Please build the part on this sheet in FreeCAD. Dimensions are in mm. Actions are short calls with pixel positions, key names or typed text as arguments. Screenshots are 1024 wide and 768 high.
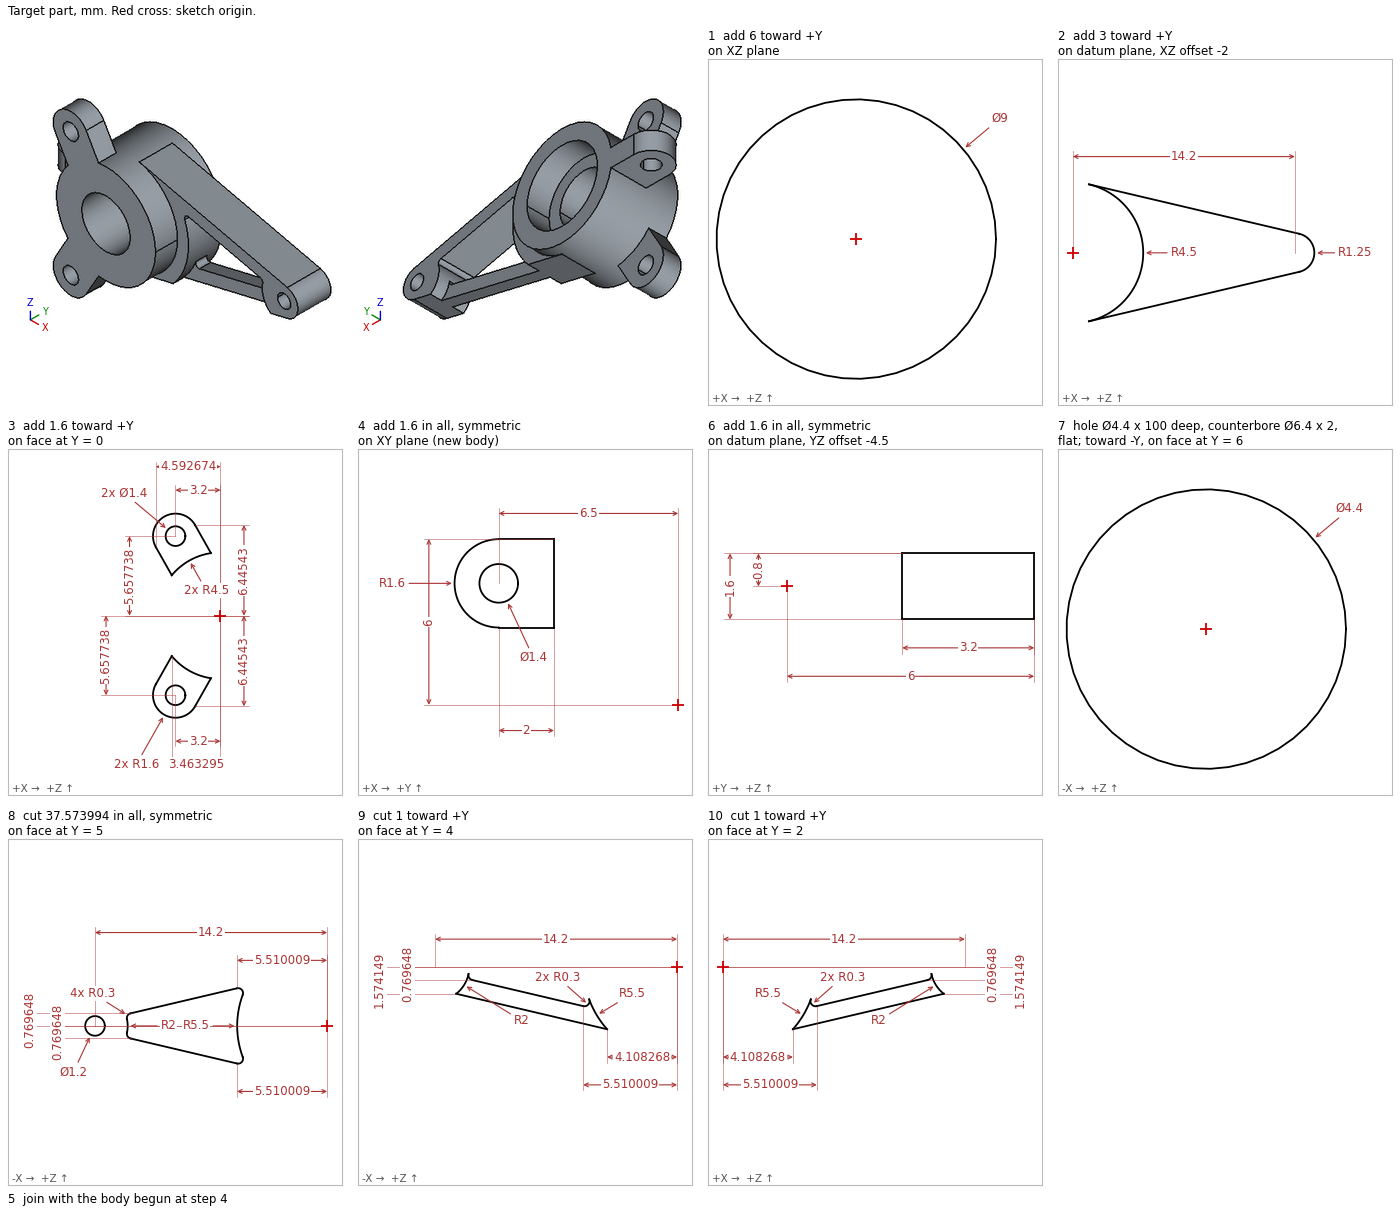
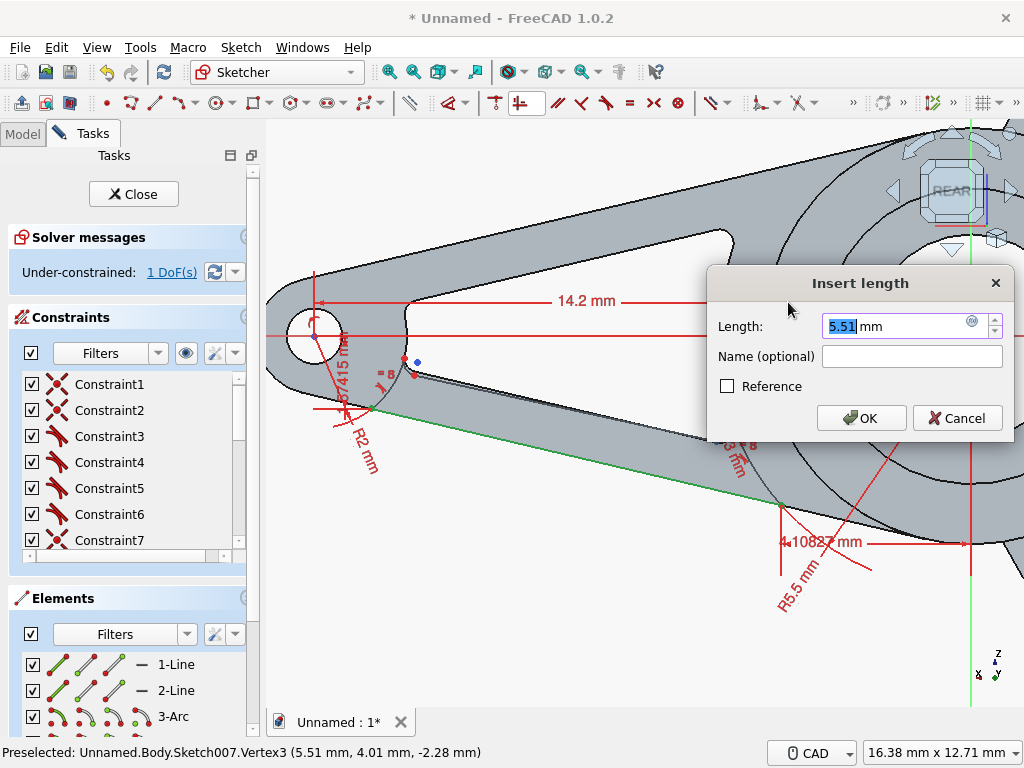
text(5.510009)
key(Return)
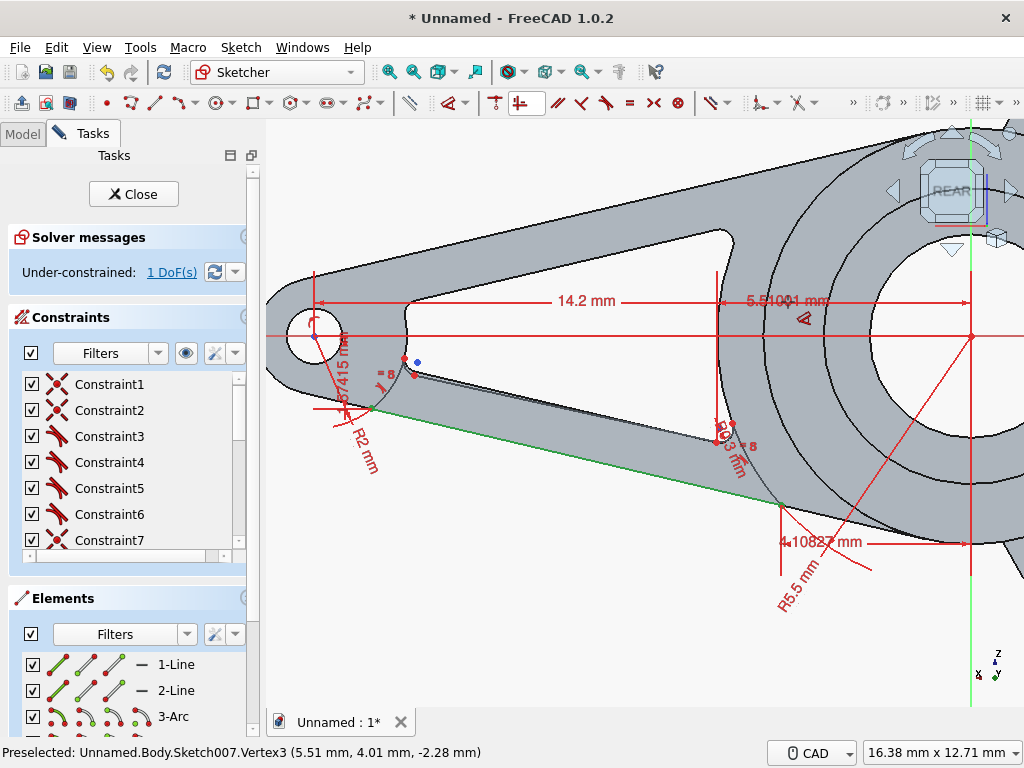
click(415, 376)
click(381, 356)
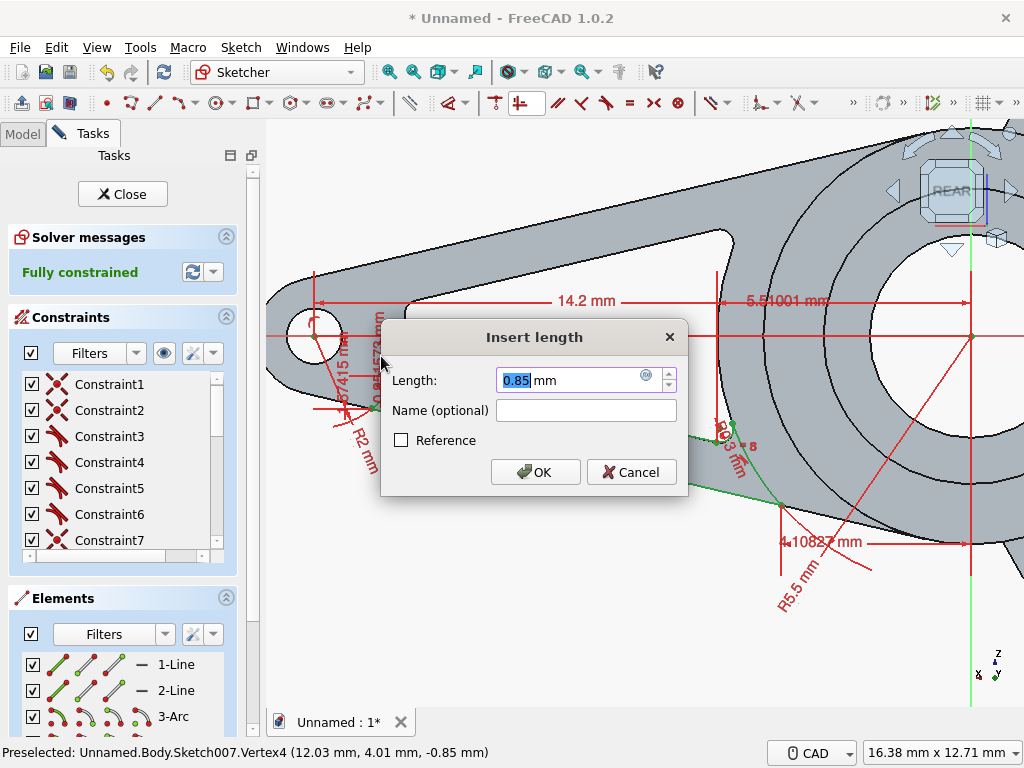
text(0.769648)
key(Return)
key(Escape)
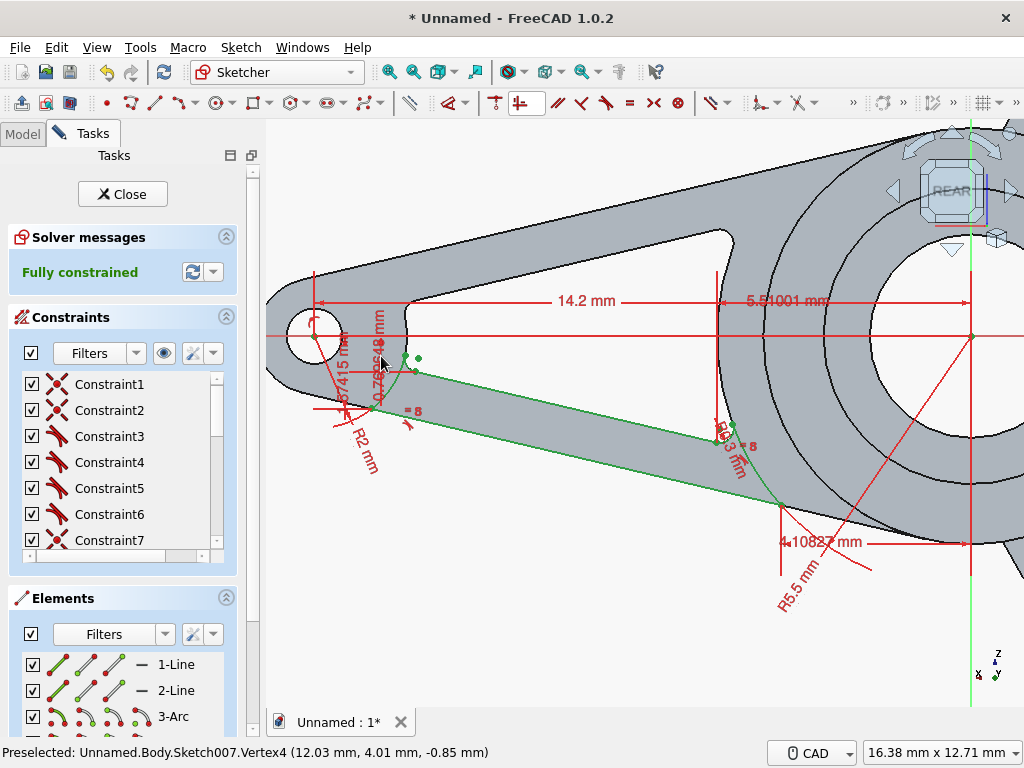
click(123, 194)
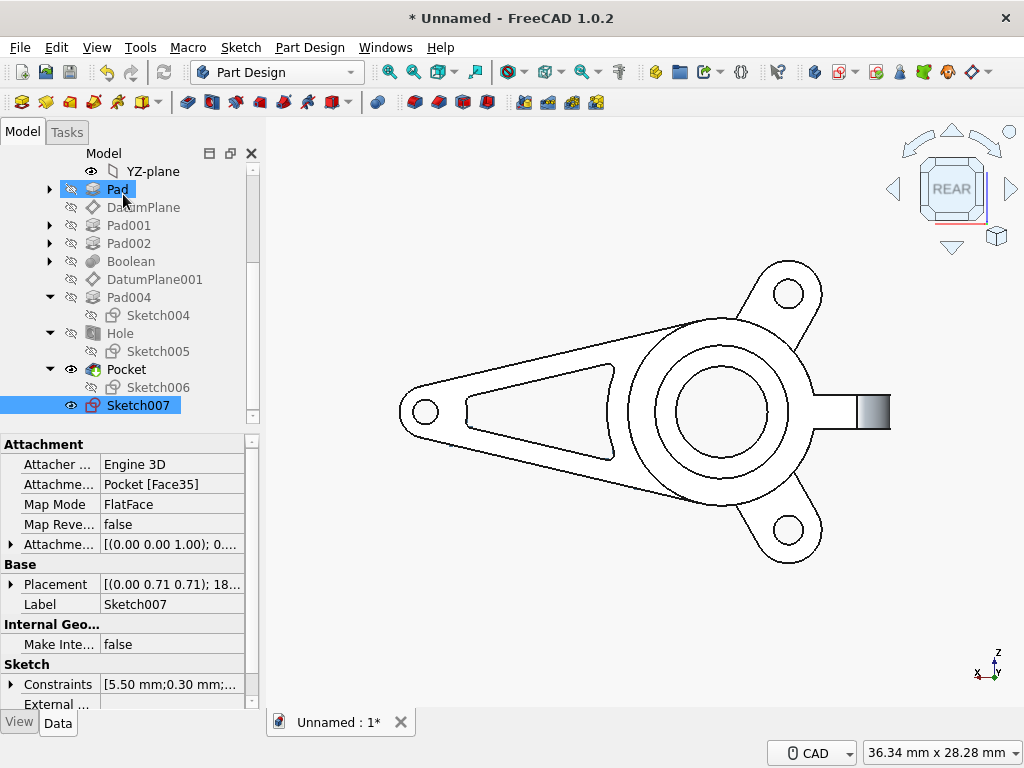
click(188, 102)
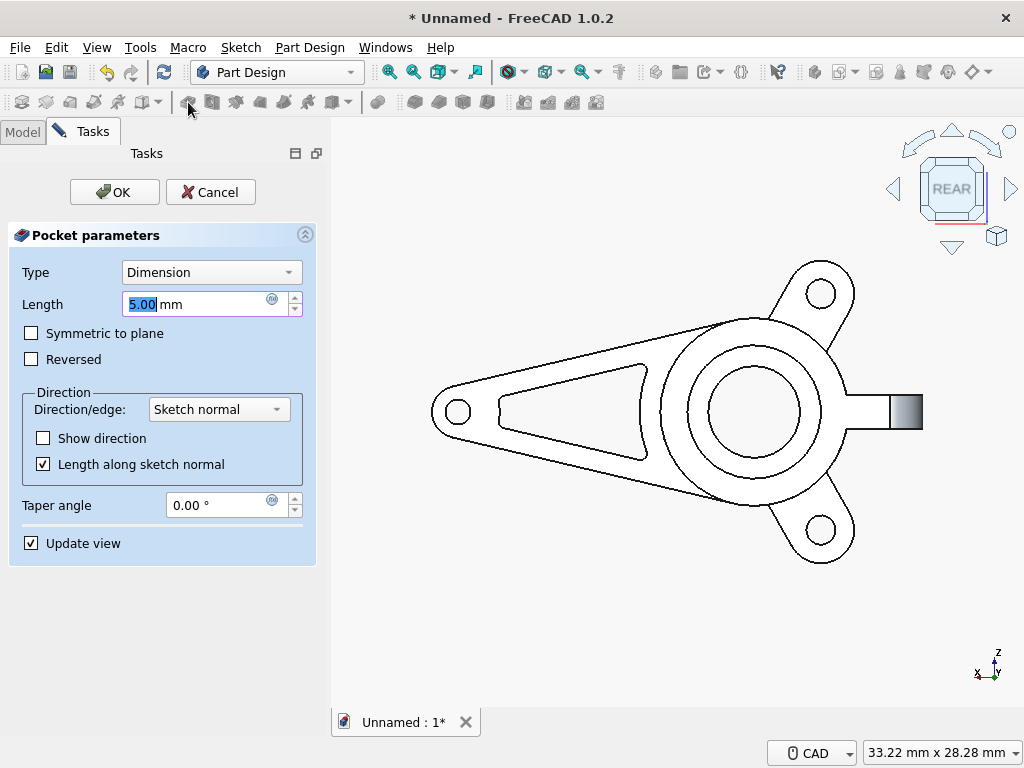
text(1)
key(Tab)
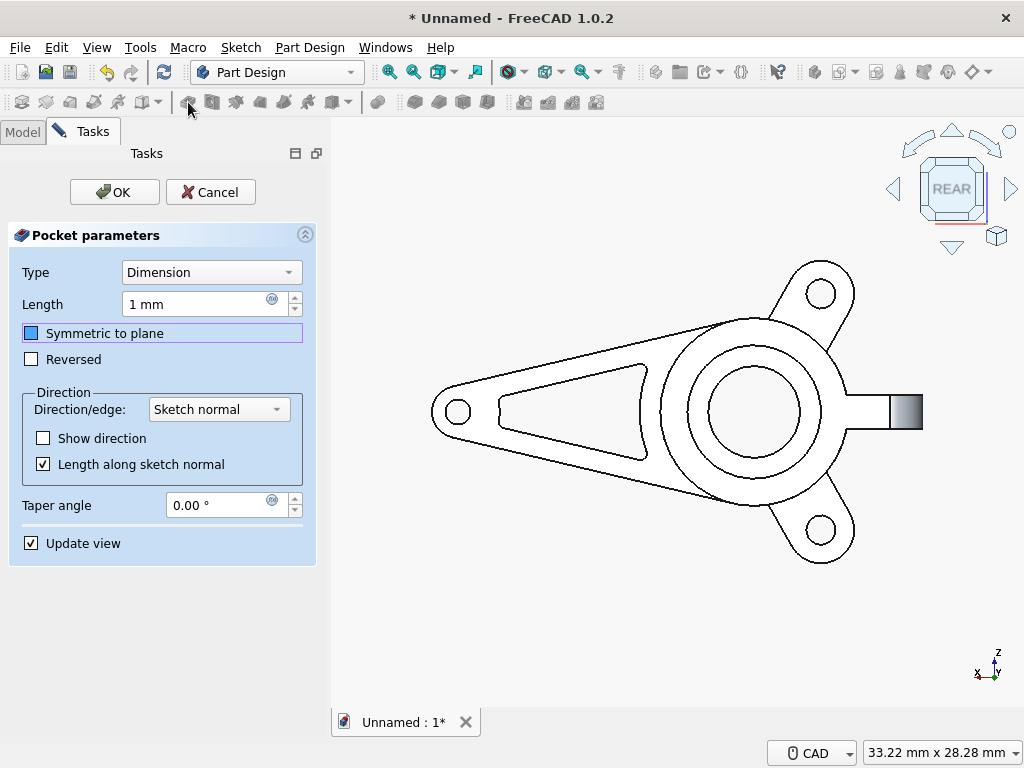
click(30, 359)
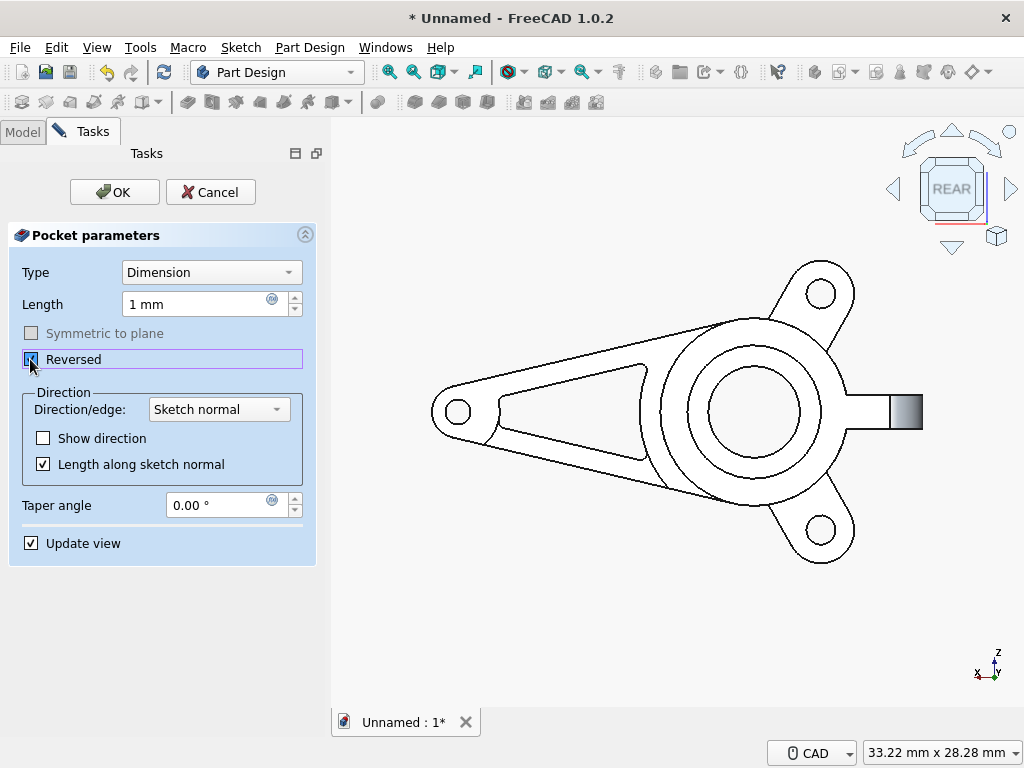
click(115, 192)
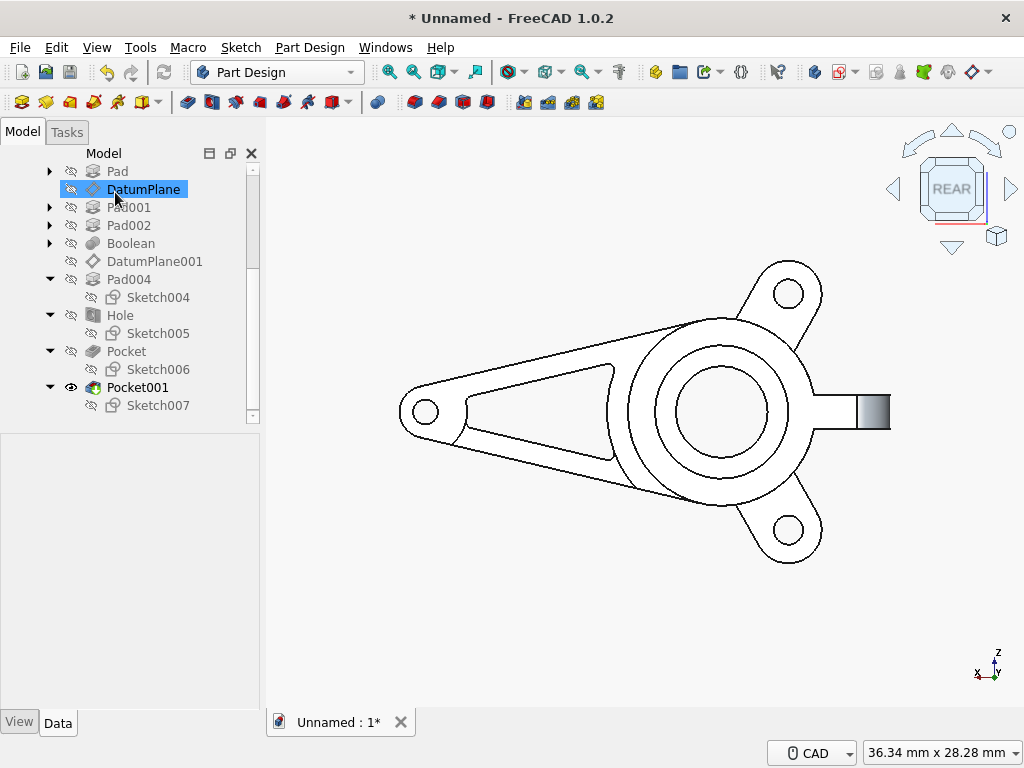
key(0)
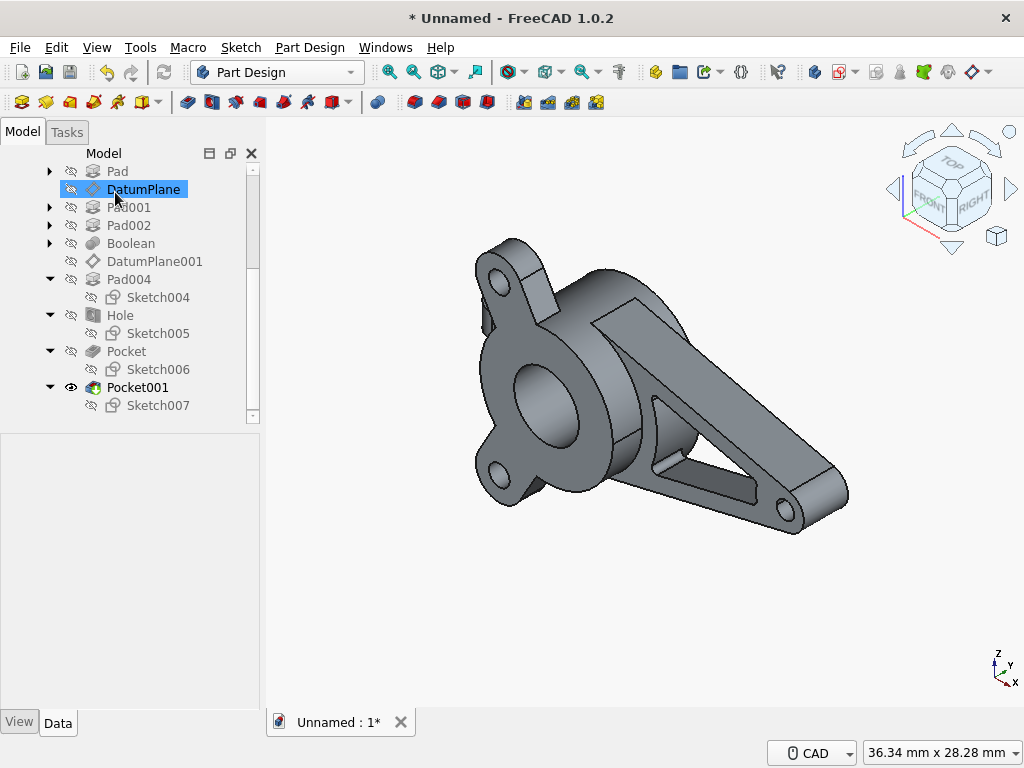
click(758, 515)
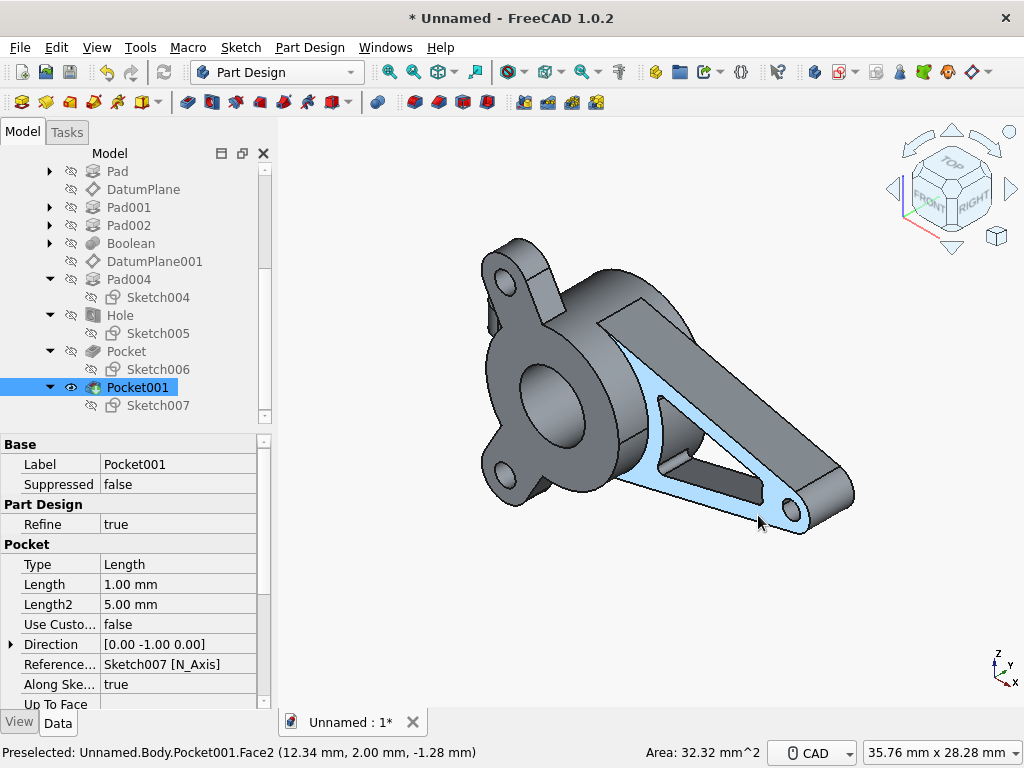
click(840, 72)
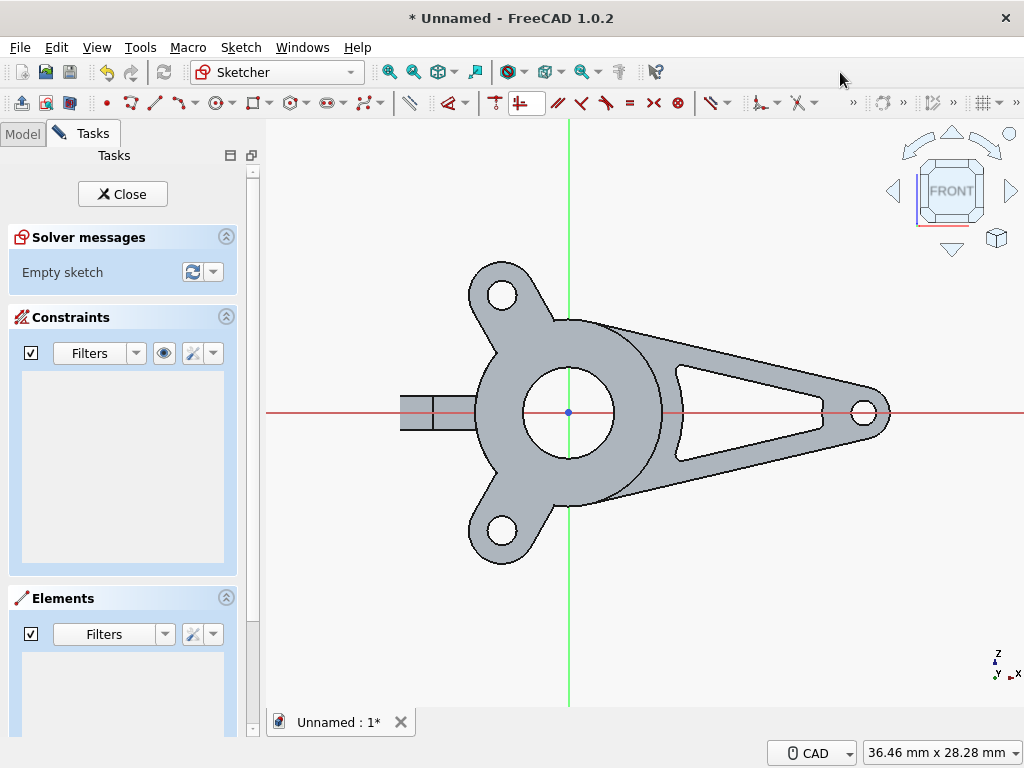
scroll(859, 528, up, 2)